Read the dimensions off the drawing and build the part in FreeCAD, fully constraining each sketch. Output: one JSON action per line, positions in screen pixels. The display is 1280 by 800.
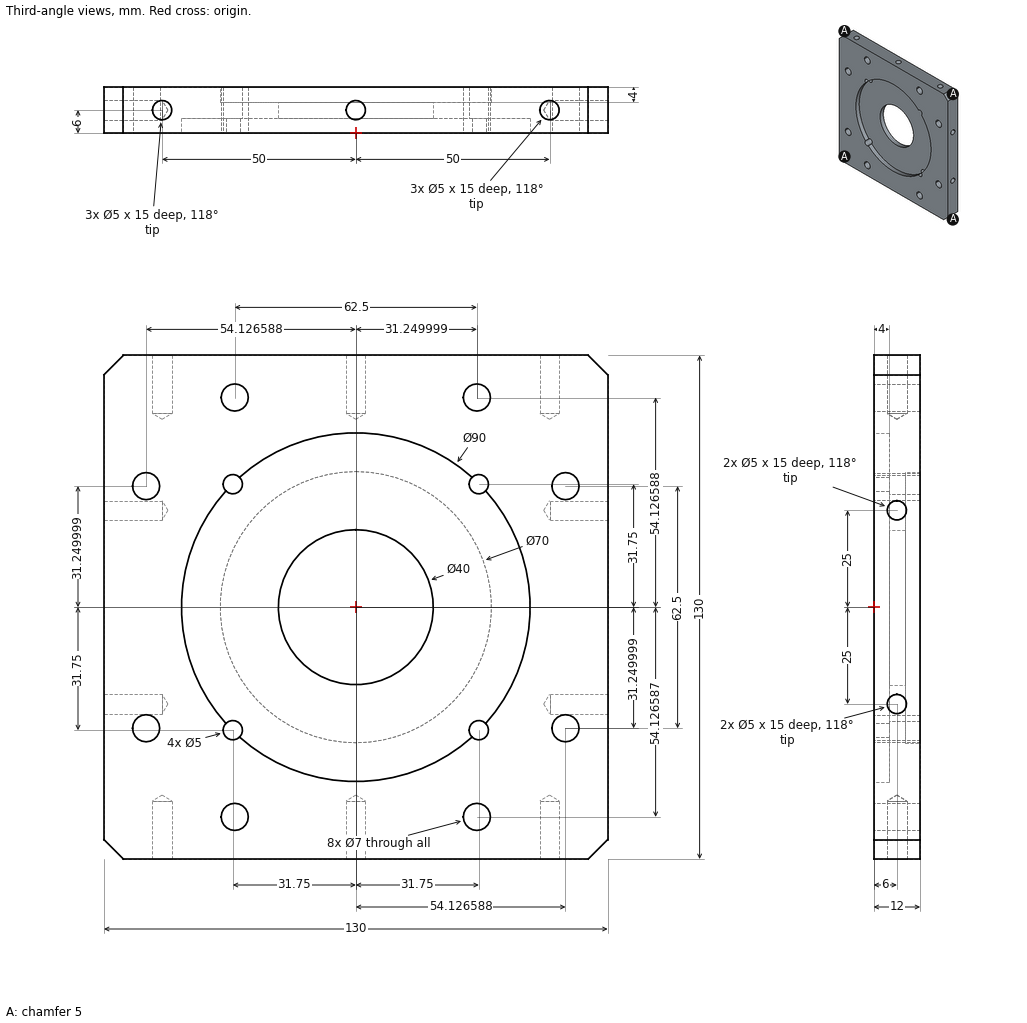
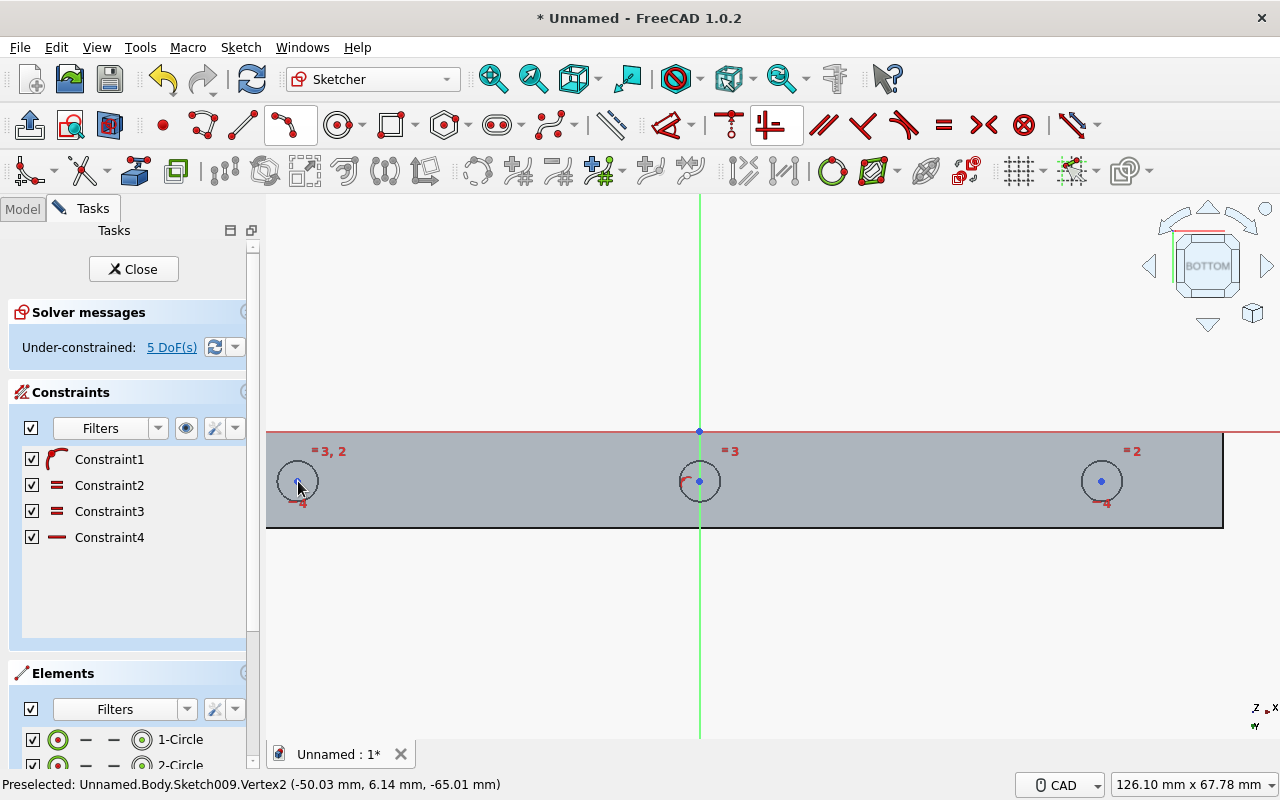
{"action": "left_click", "coordinate": [1102, 481]}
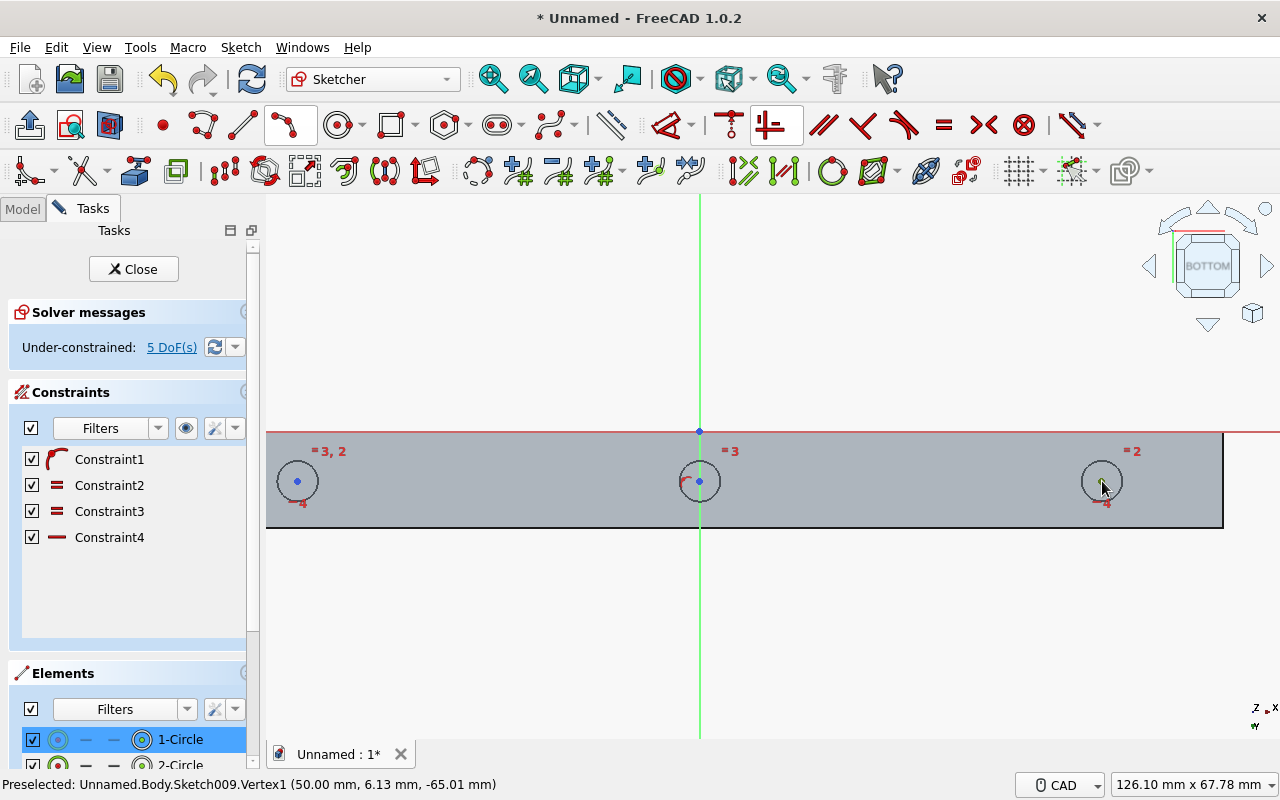
{"action": "left_click", "coordinate": [700, 481]}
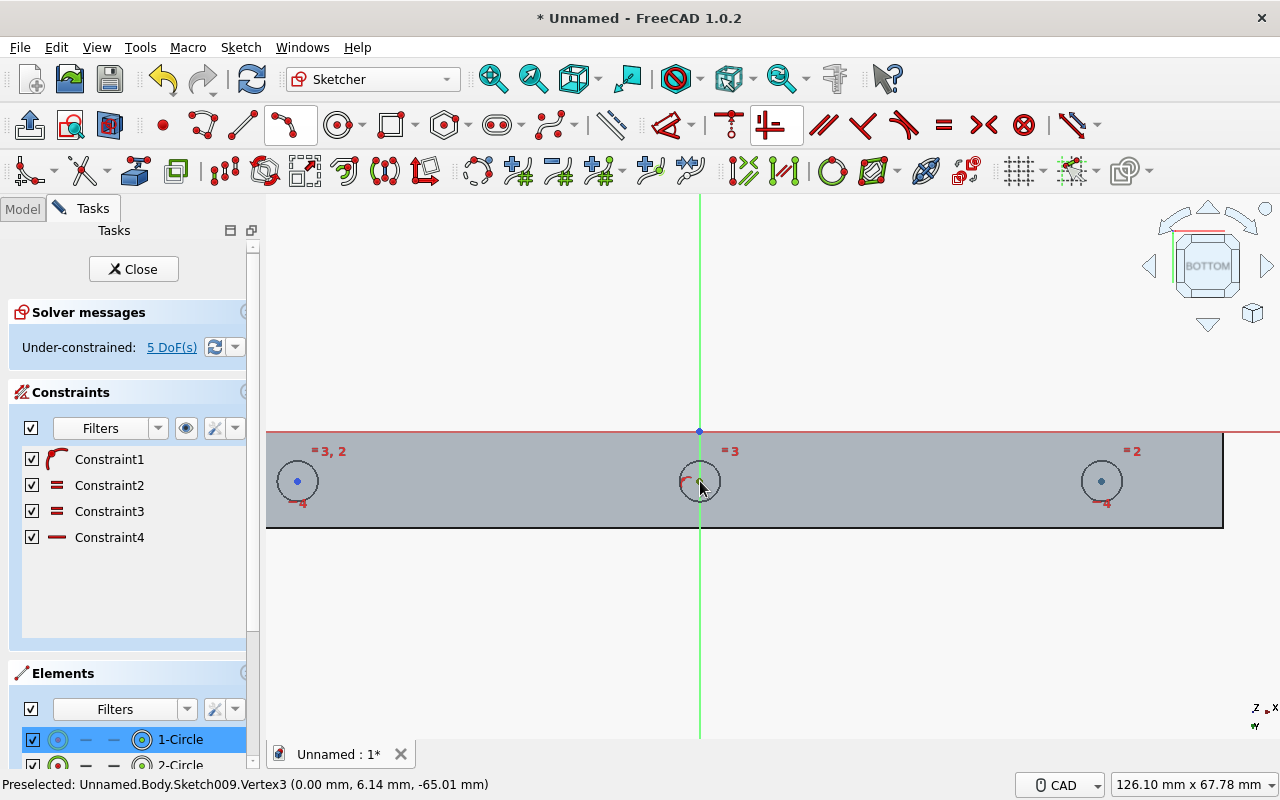
{"action": "key", "text": "h"}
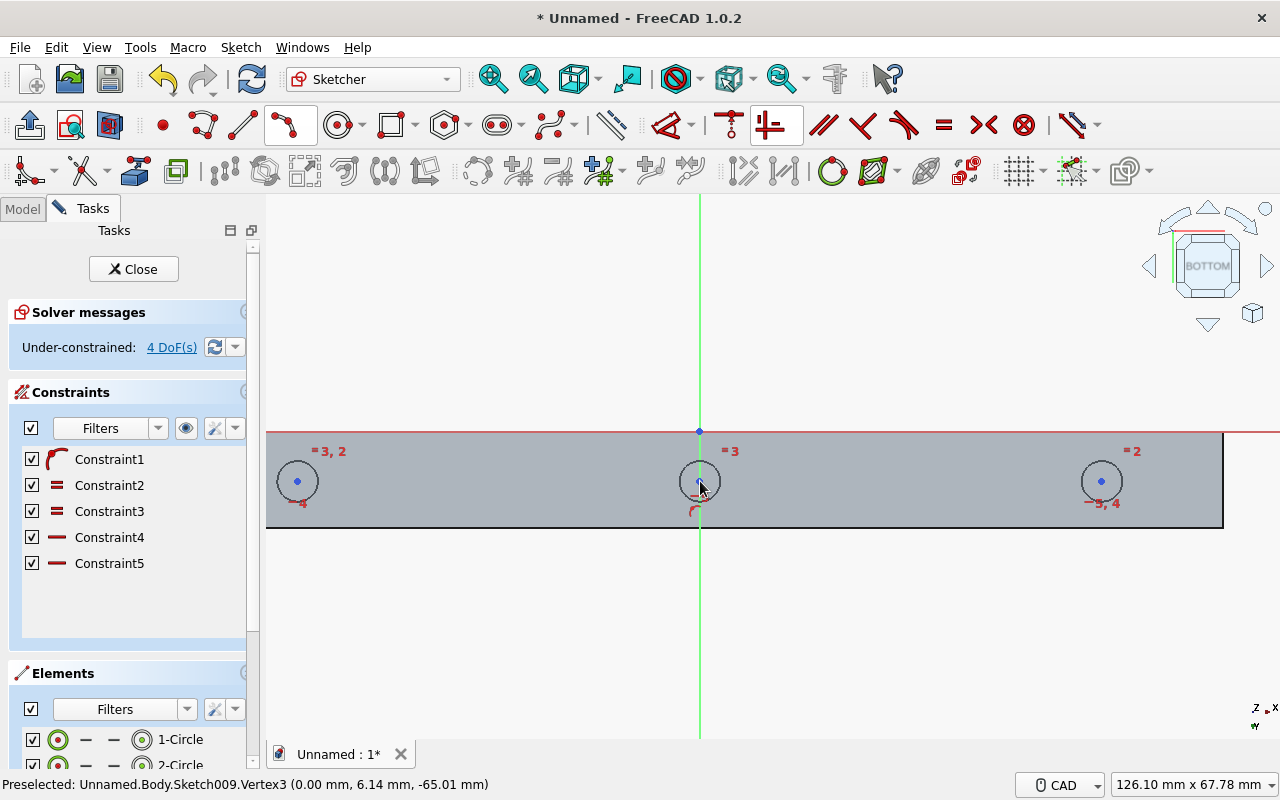
{"action": "key", "text": "d"}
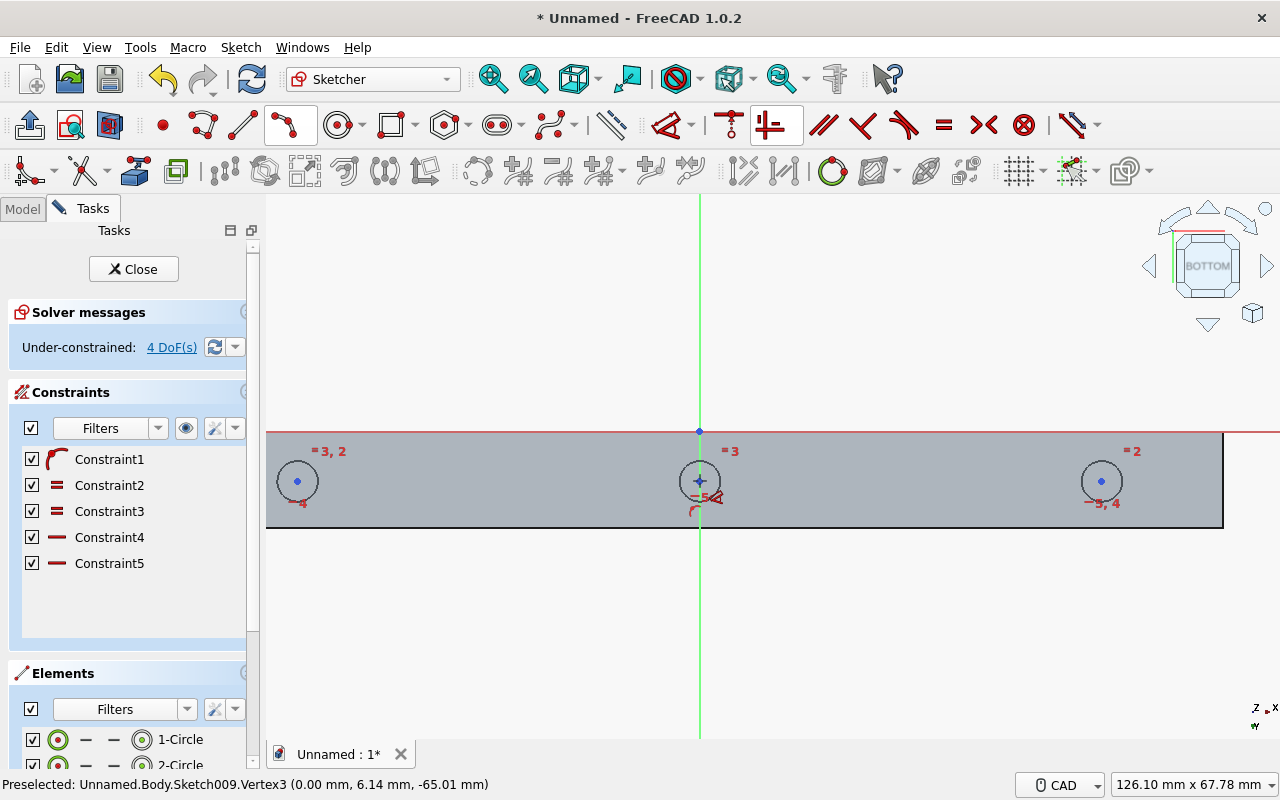
{"action": "left_click", "coordinate": [1088, 467]}
{"action": "left_click", "coordinate": [1052, 466]}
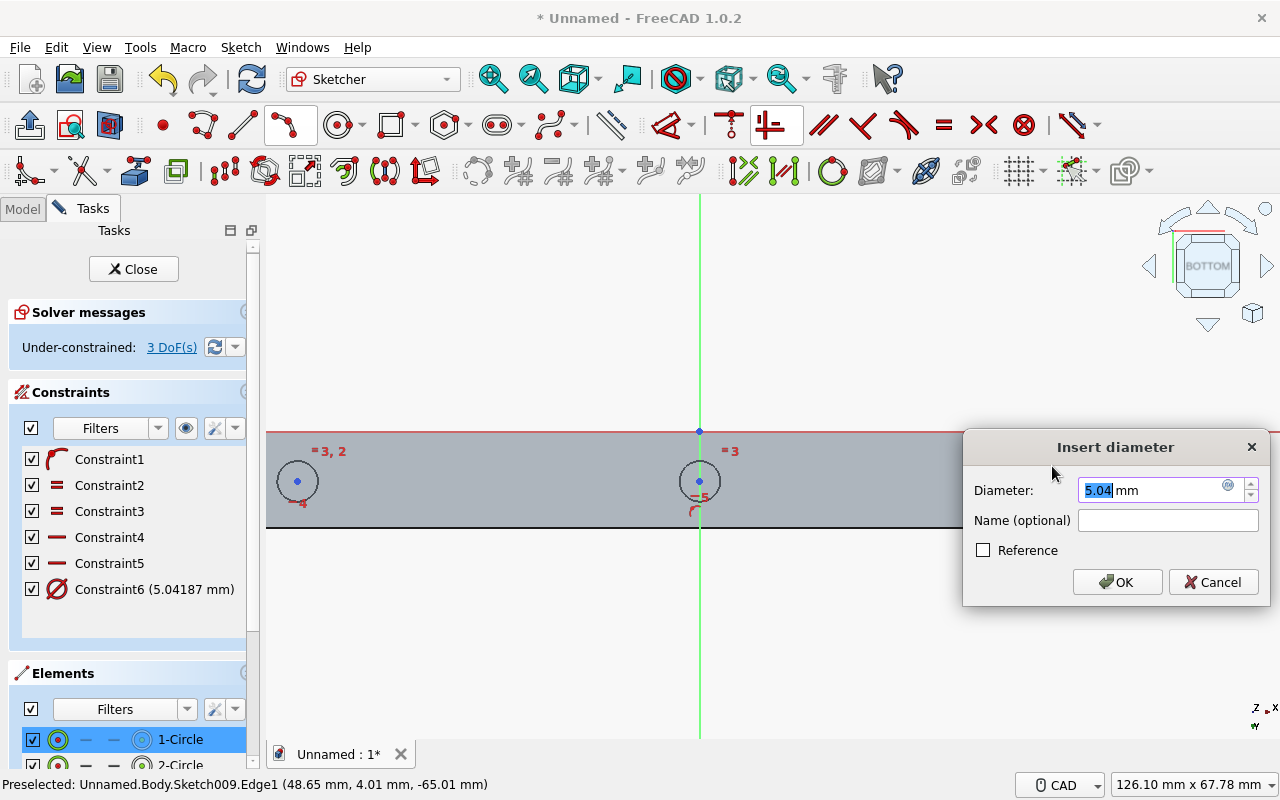
{"action": "type", "text": "5"}
{"action": "key", "text": "Return"}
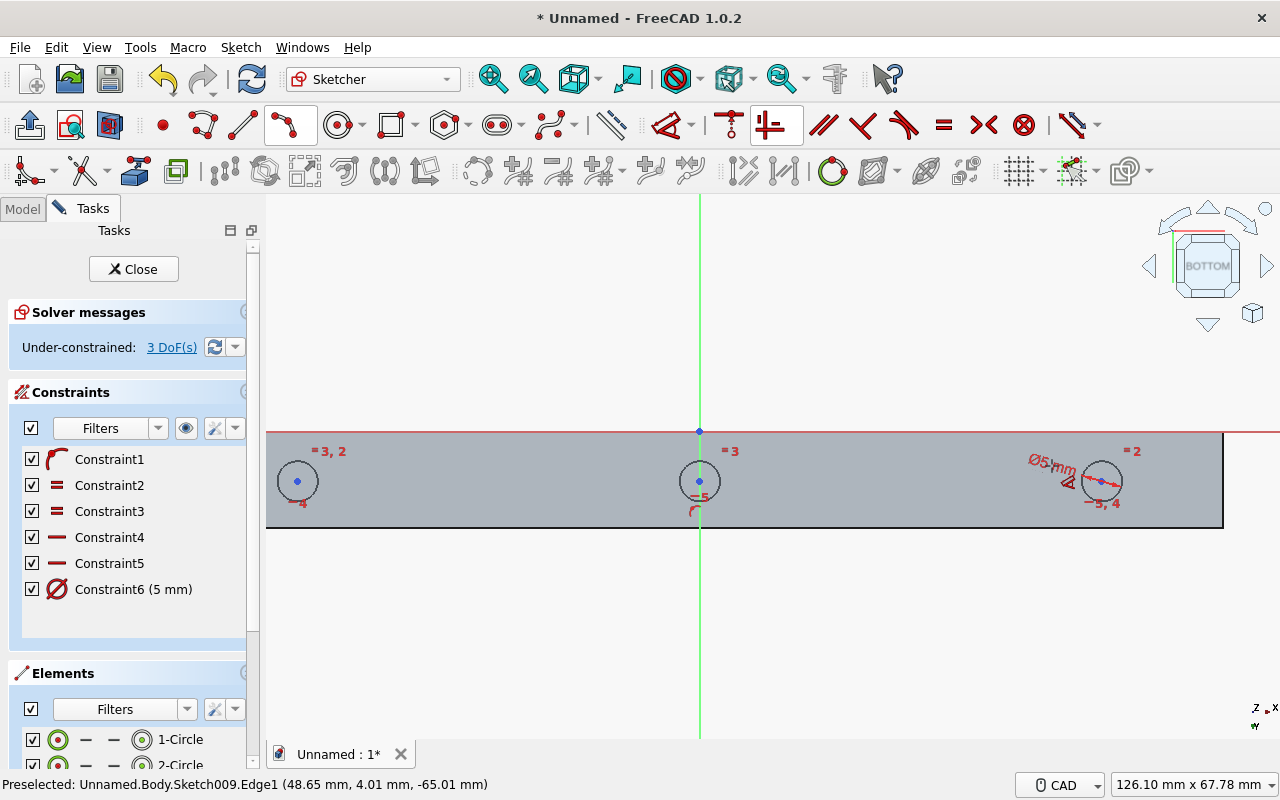
{"action": "left_click", "coordinate": [1102, 481]}
{"action": "left_click", "coordinate": [666, 457]}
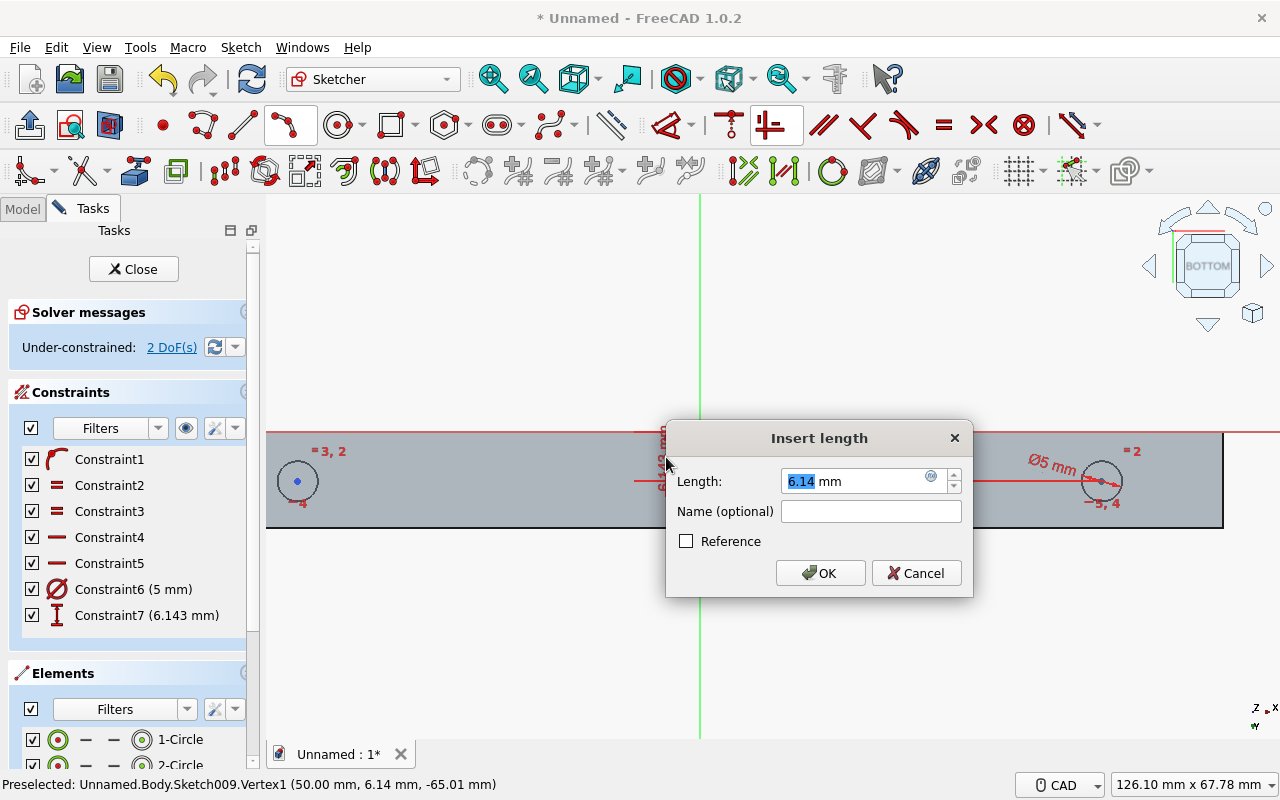
{"action": "type", "text": "6"}
{"action": "key", "text": "Return"}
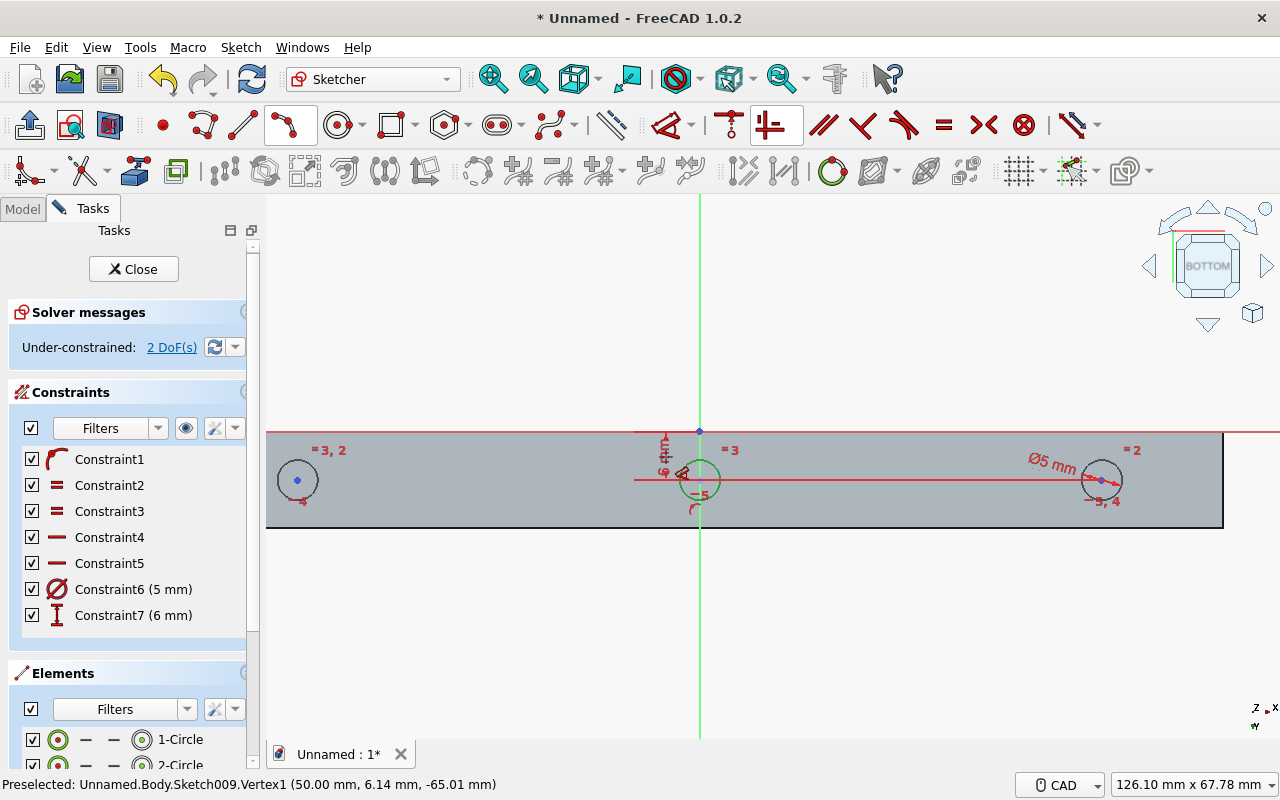
{"action": "left_click", "coordinate": [1102, 480]}
{"action": "left_click", "coordinate": [901, 398]}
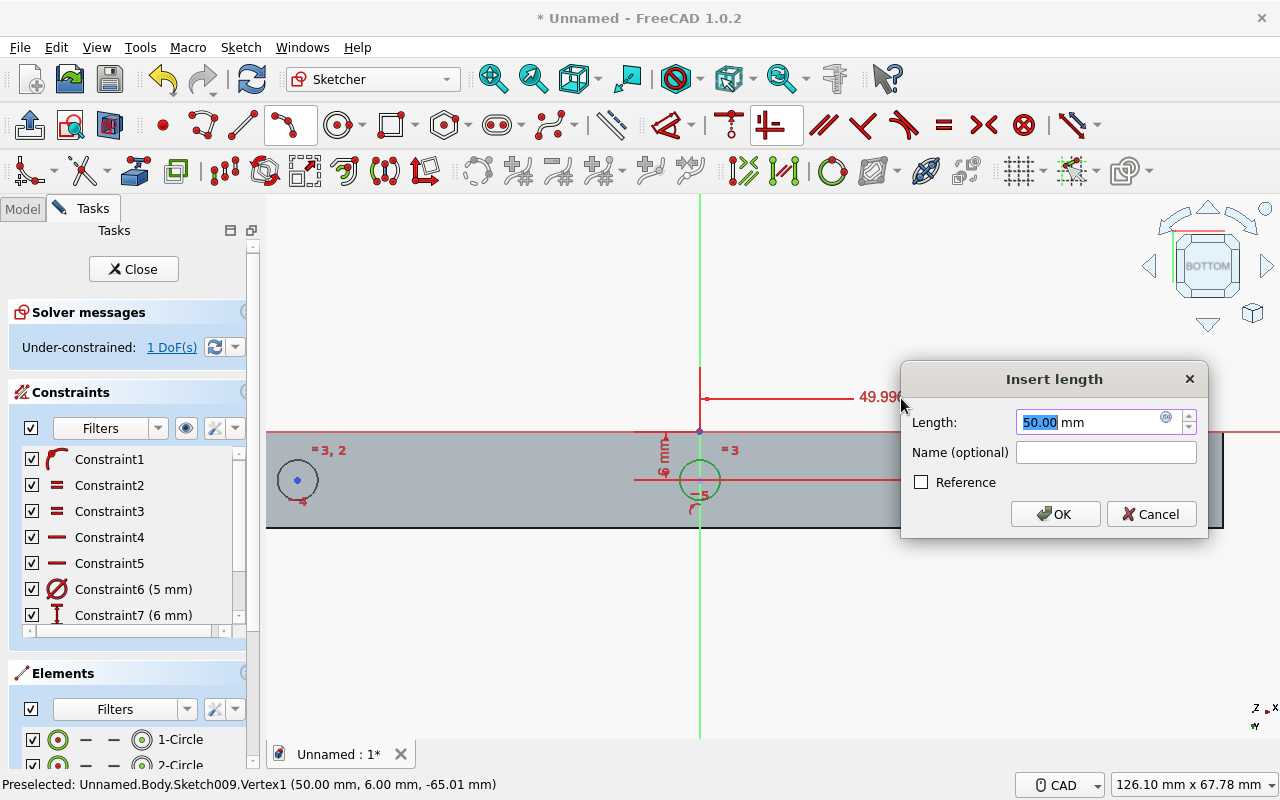
{"action": "type", "text": "50"}
{"action": "key", "text": "Return"}